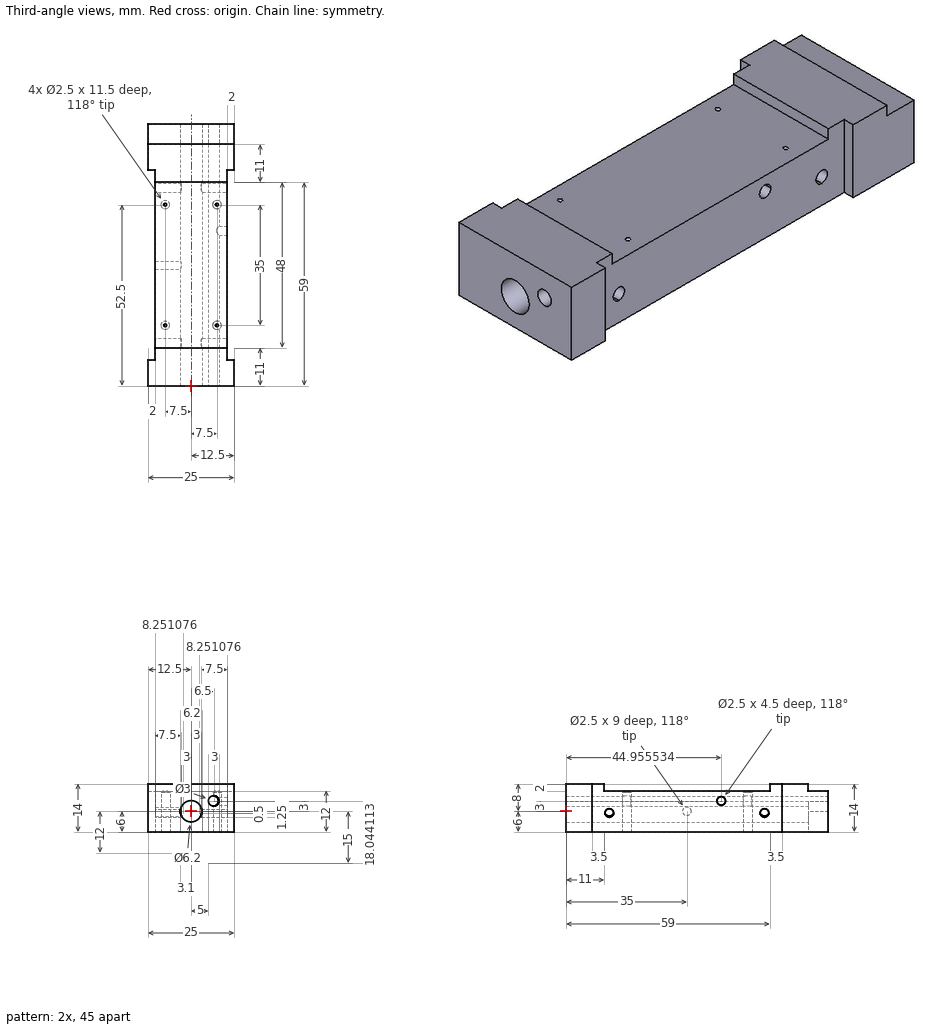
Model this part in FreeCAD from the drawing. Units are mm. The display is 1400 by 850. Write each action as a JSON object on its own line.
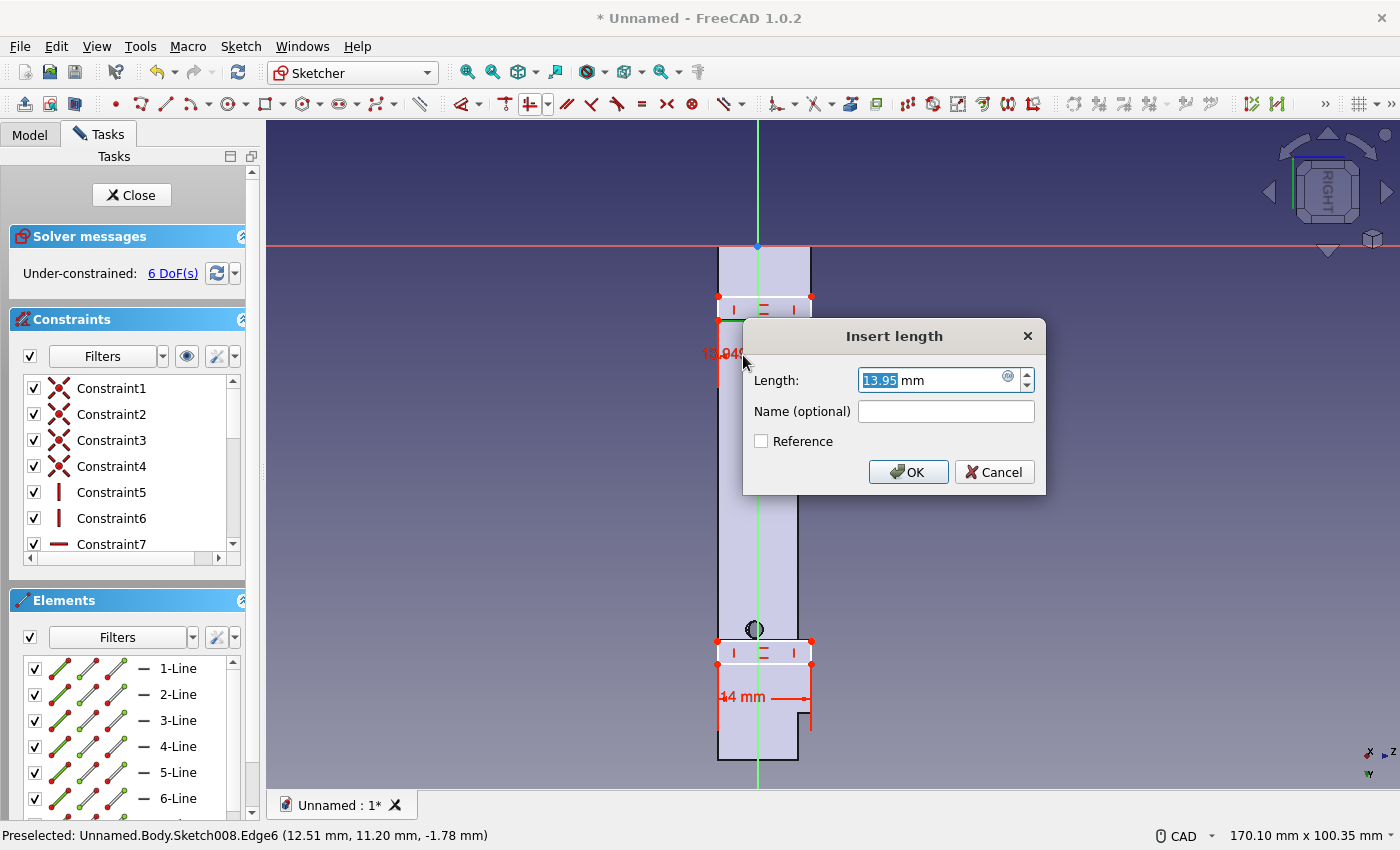
{"action": "type", "text": "14"}
{"action": "key", "text": "Return"}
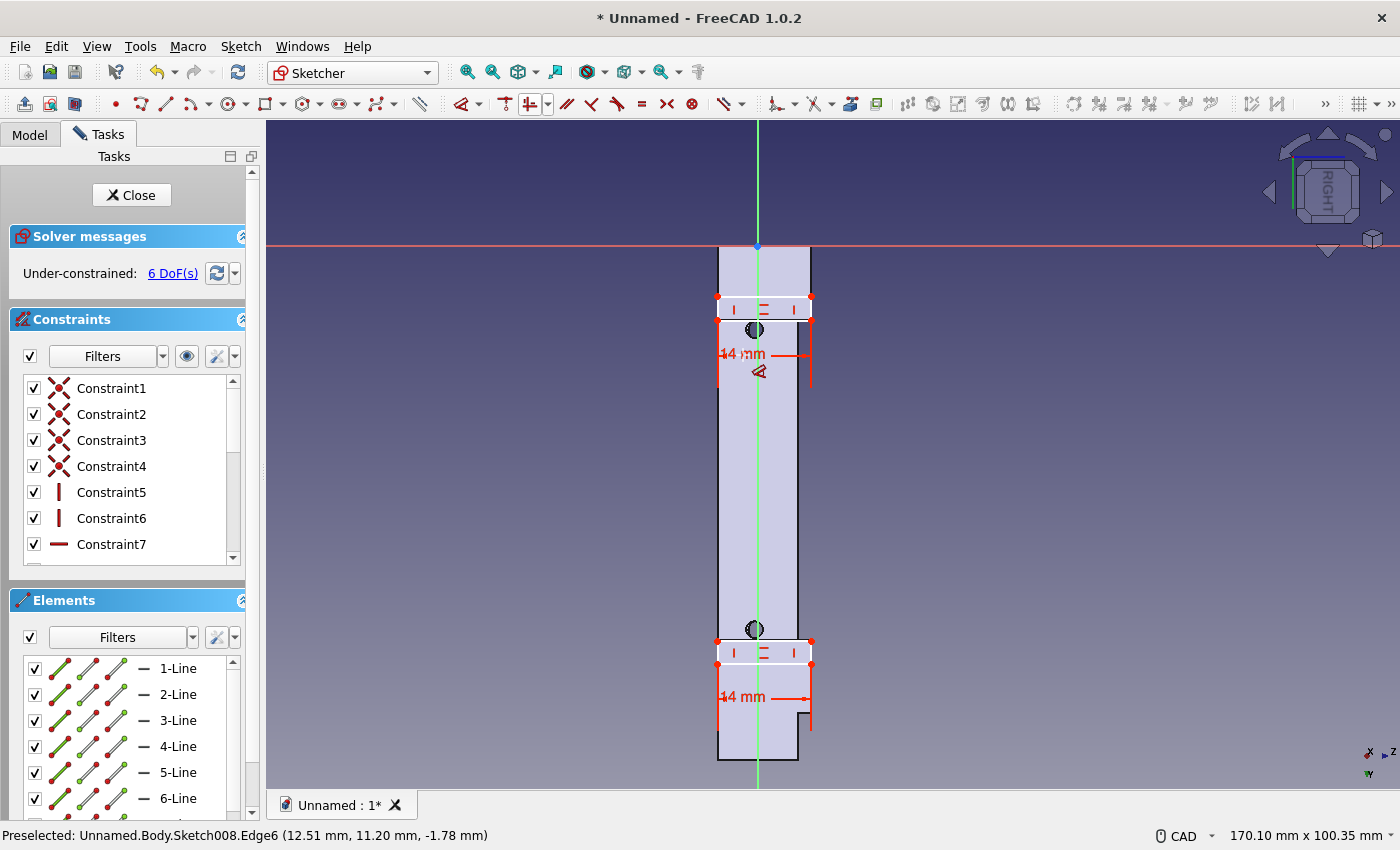
{"action": "left_click", "coordinate": [718, 641]}
{"action": "left_click", "coordinate": [738, 212]}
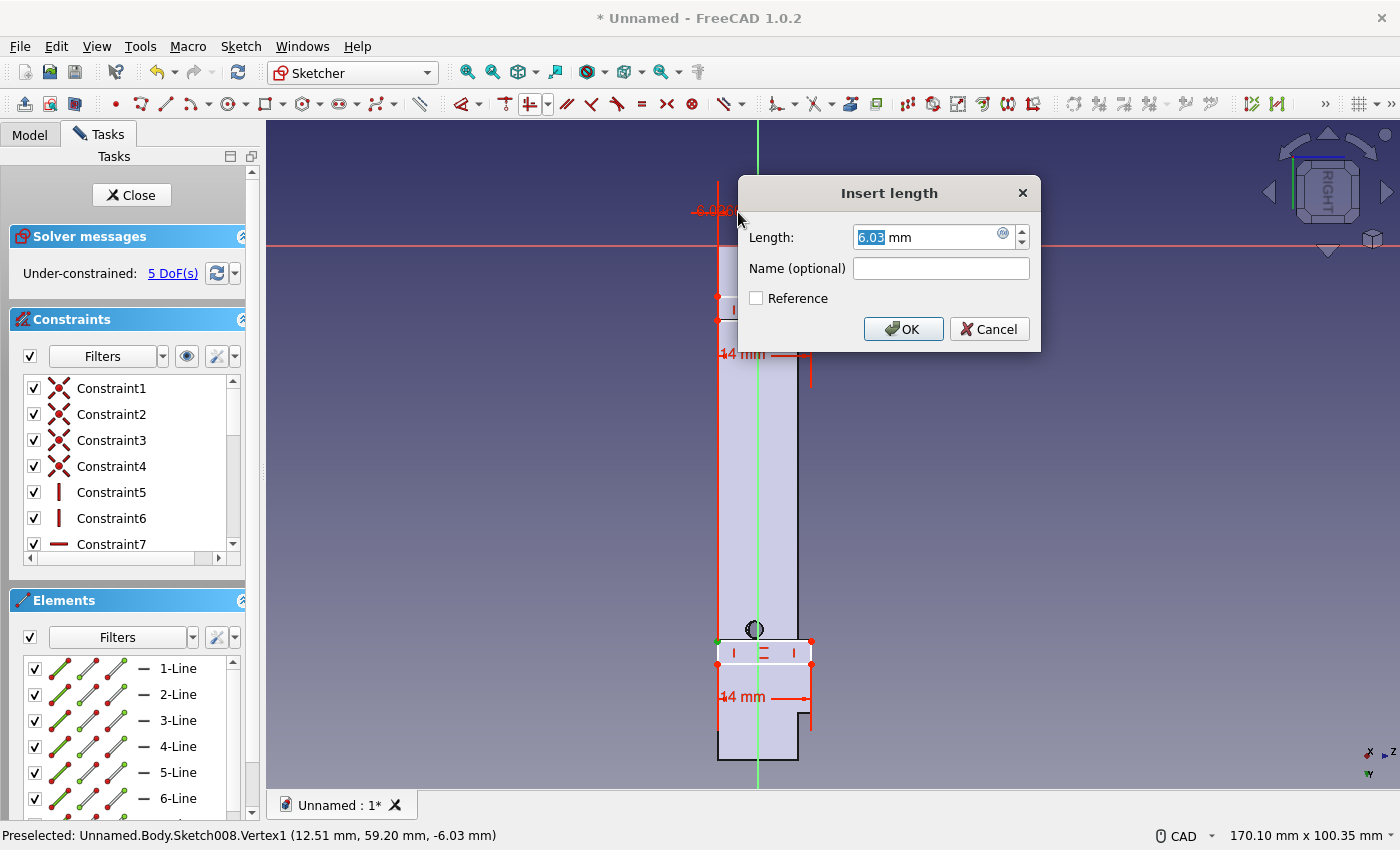
{"action": "type", "text": "6"}
{"action": "key", "text": "Return"}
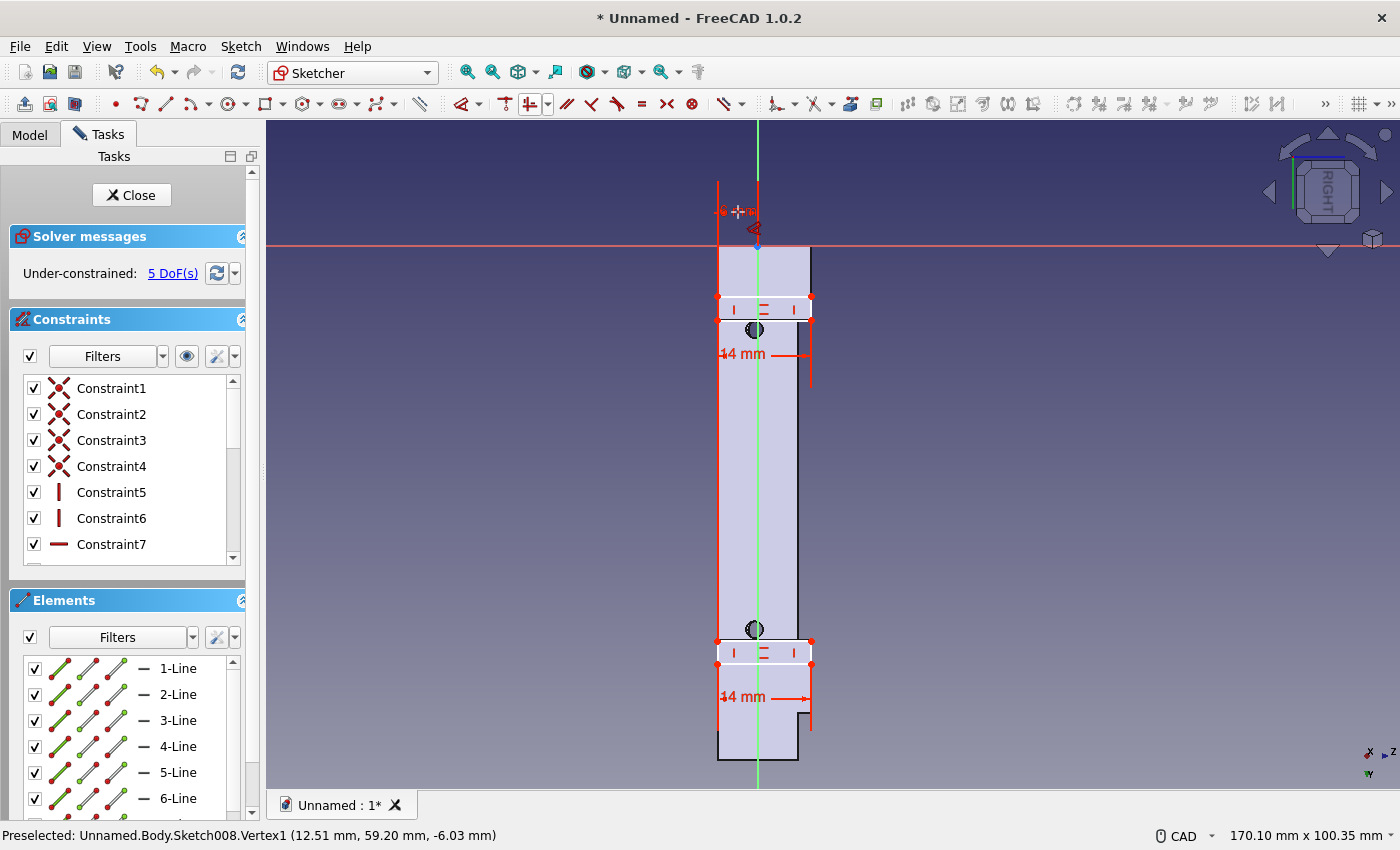
{"action": "left_click", "coordinate": [718, 297]}
{"action": "left_click", "coordinate": [738, 188]}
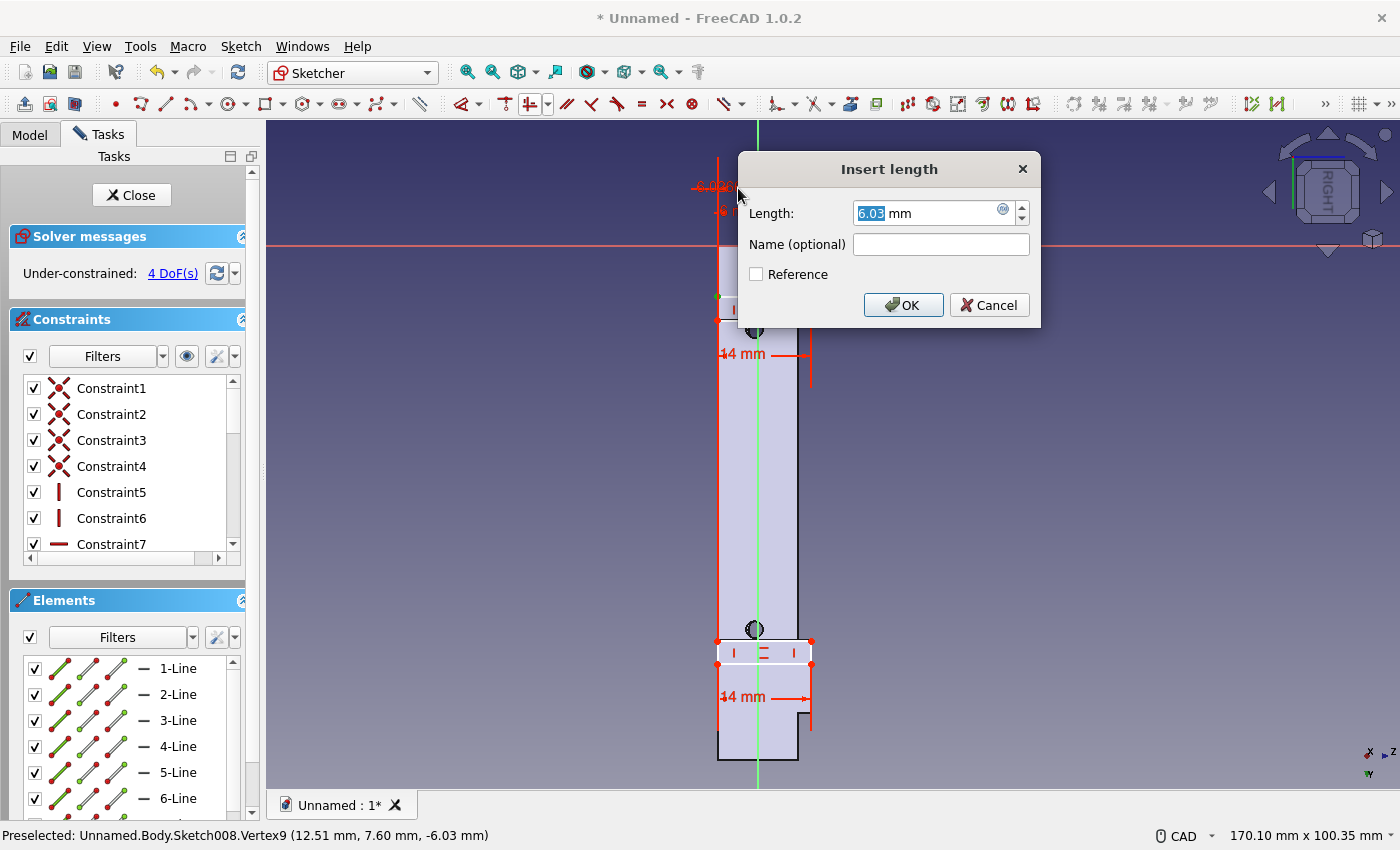
{"action": "type", "text": "6"}
{"action": "key", "text": "Return"}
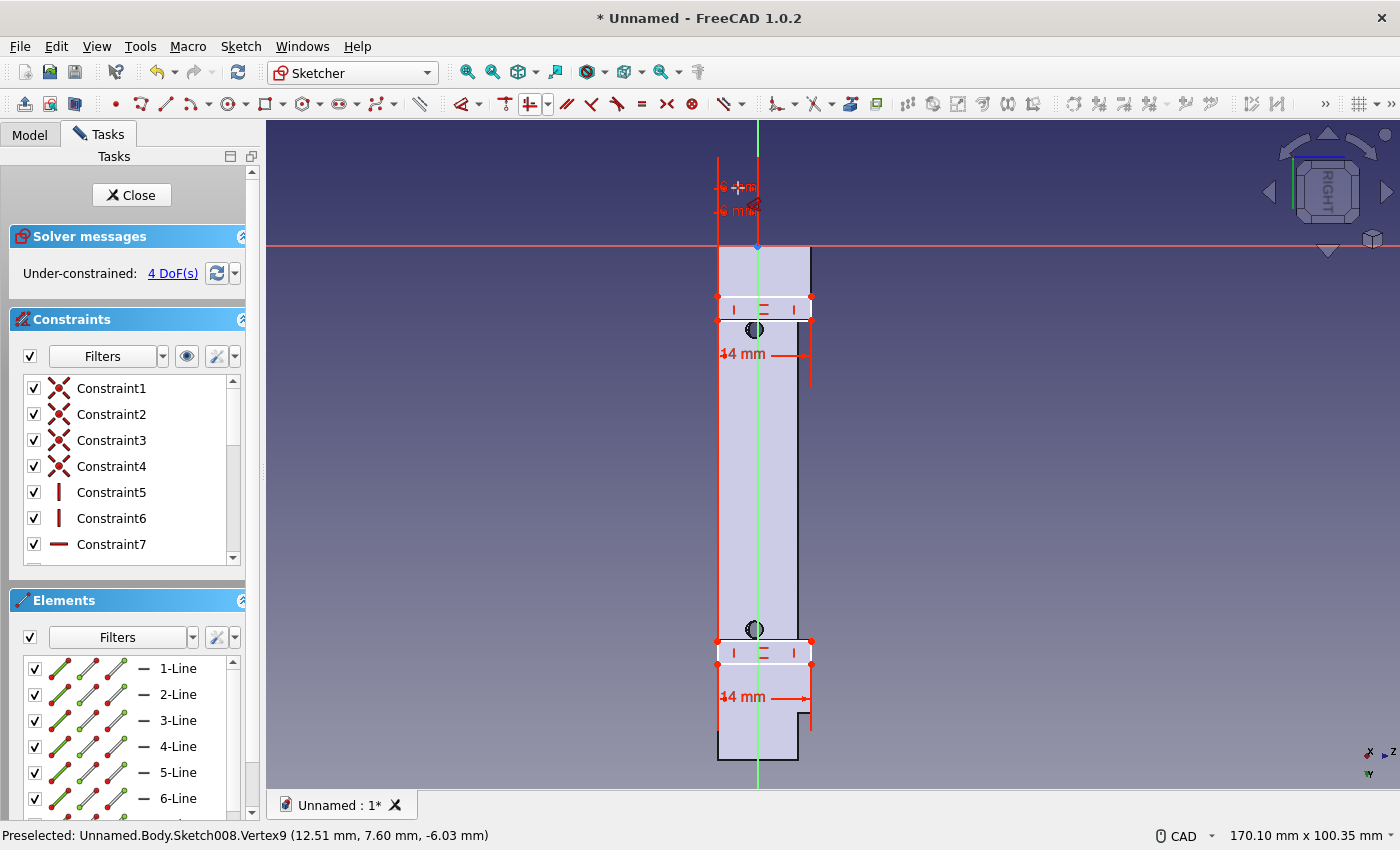
{"action": "scroll", "coordinate": [718, 650], "scroll_direction": "up", "scroll_amount": 3}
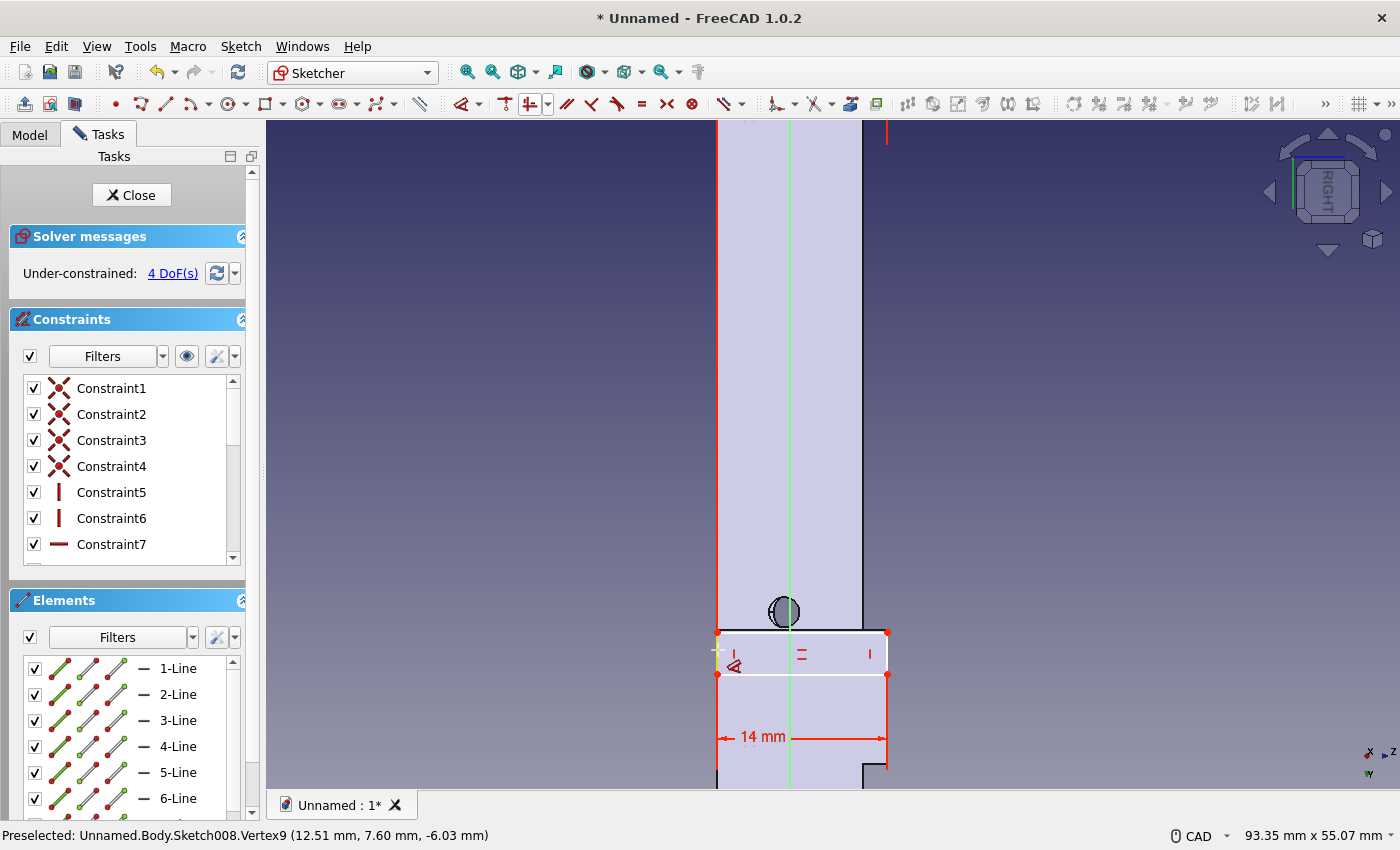
{"action": "left_click", "coordinate": [717, 650]}
{"action": "left_click", "coordinate": [683, 654]}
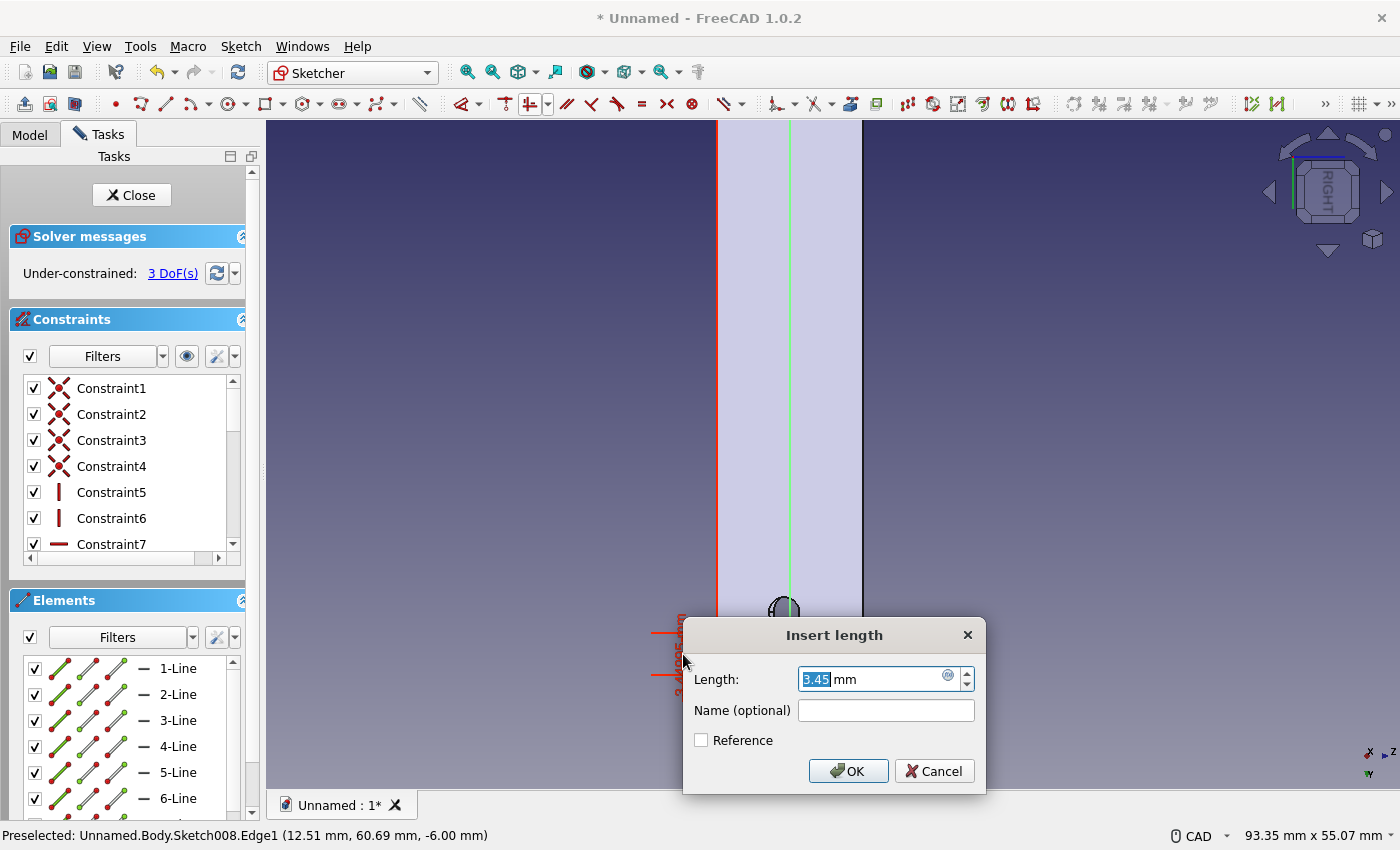
{"action": "type", "text": "3.5"}
{"action": "key", "text": "Return"}